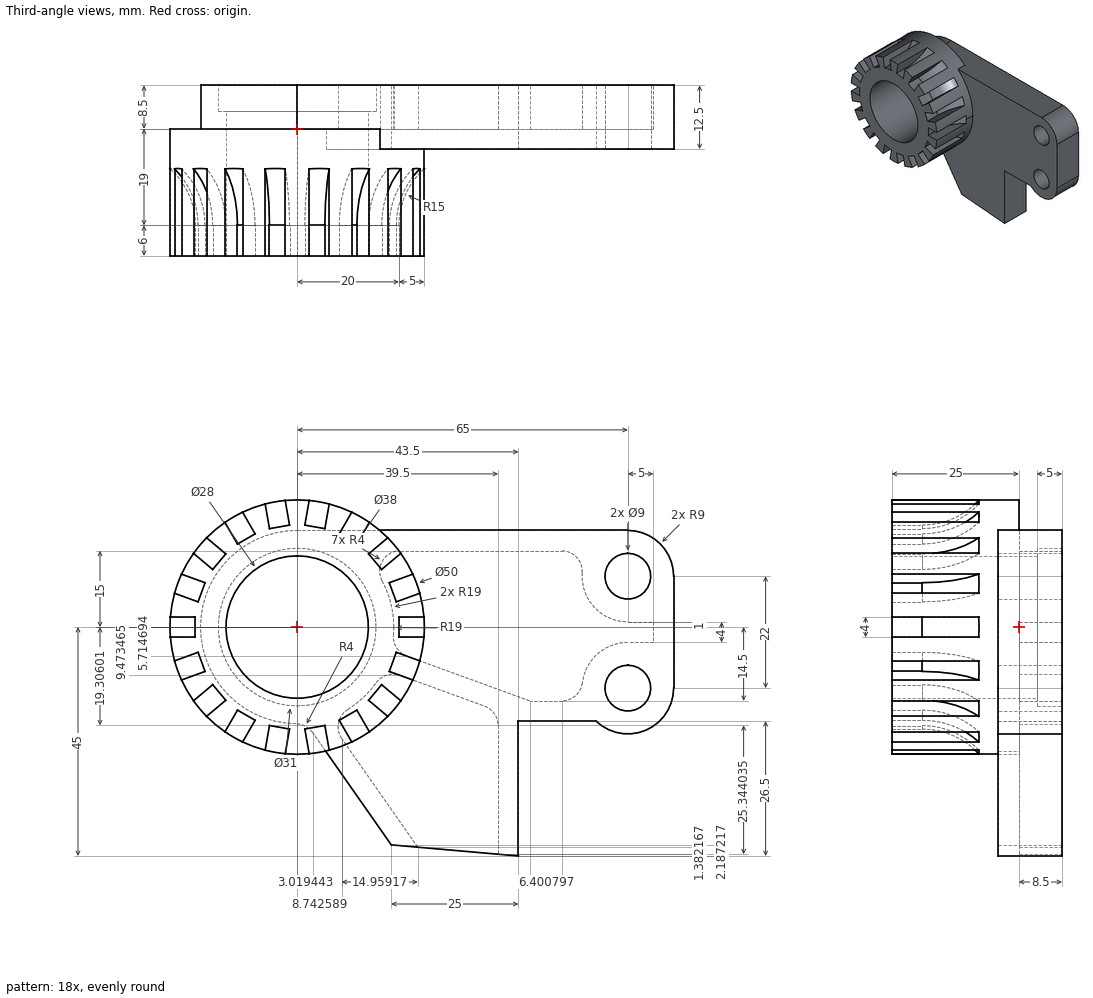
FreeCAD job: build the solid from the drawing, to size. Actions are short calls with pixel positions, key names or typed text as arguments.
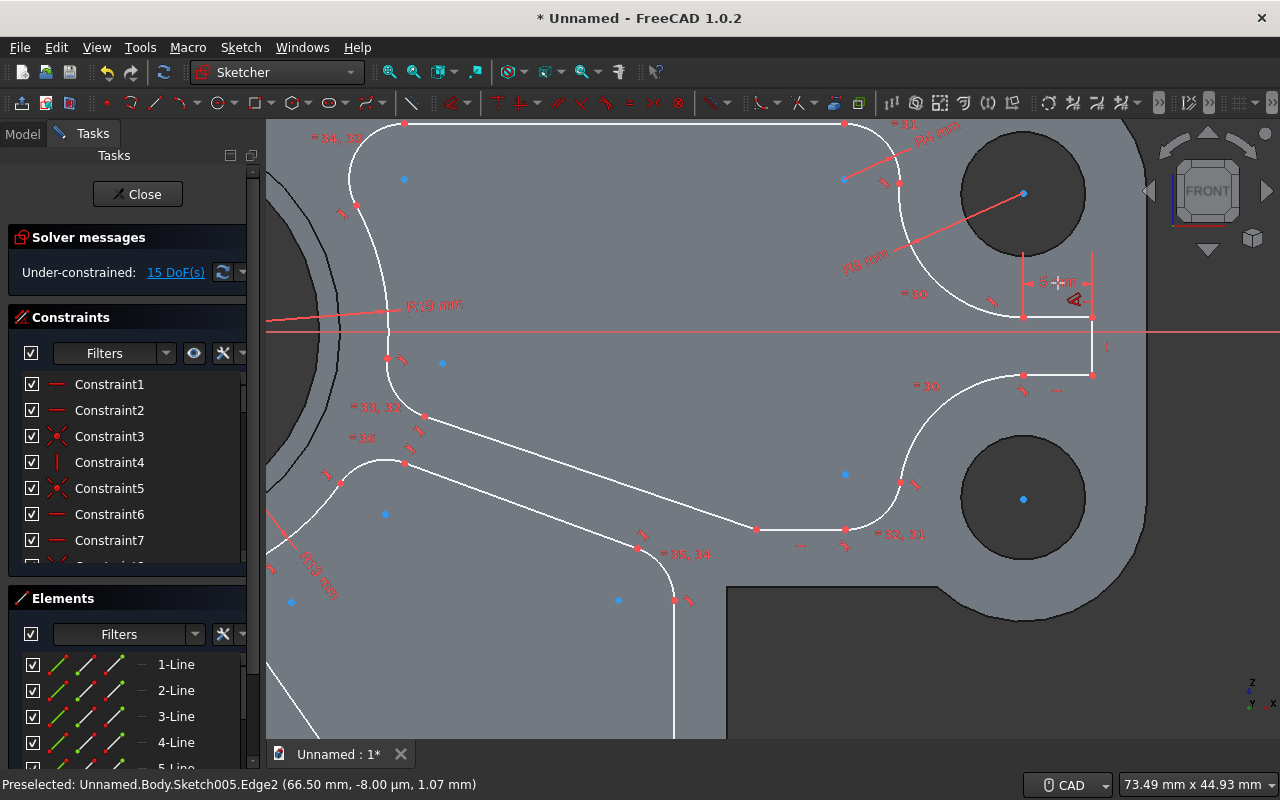
click(1092, 335)
click(1058, 346)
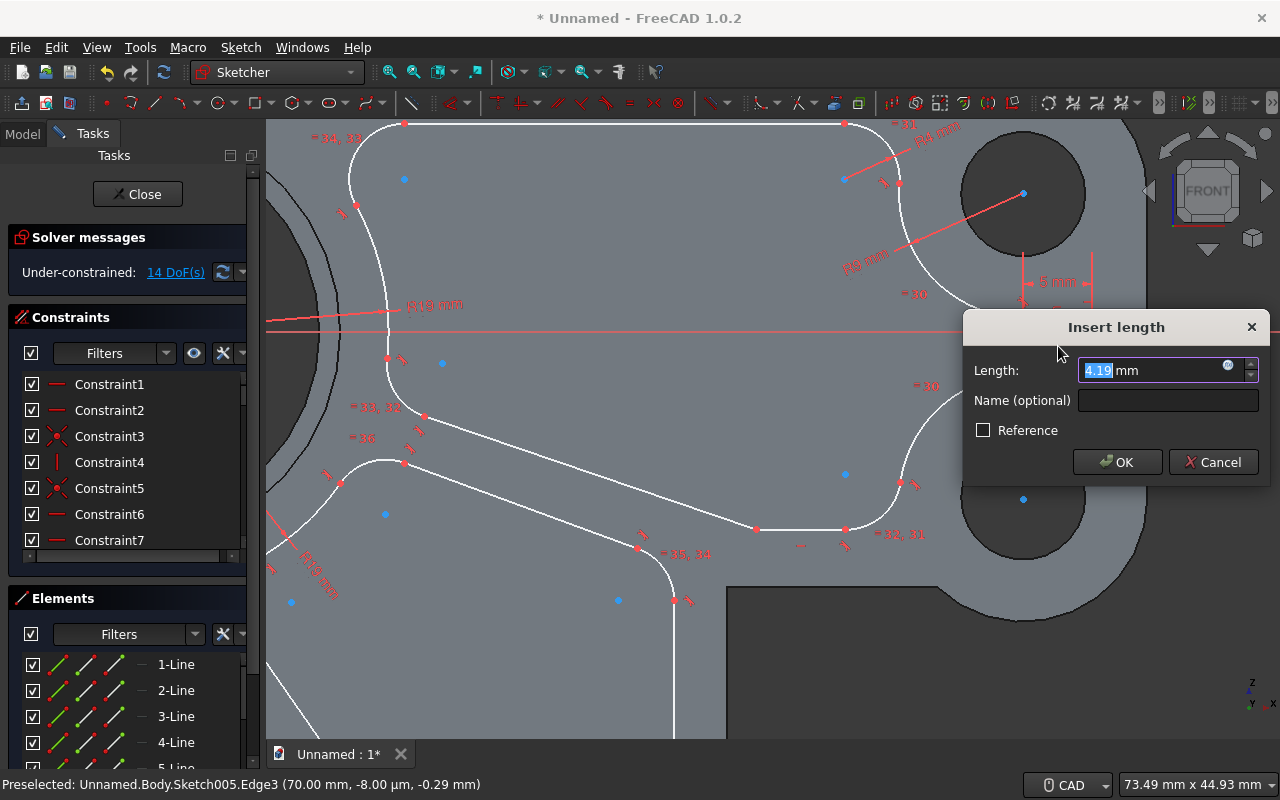
text(4)
key(Return)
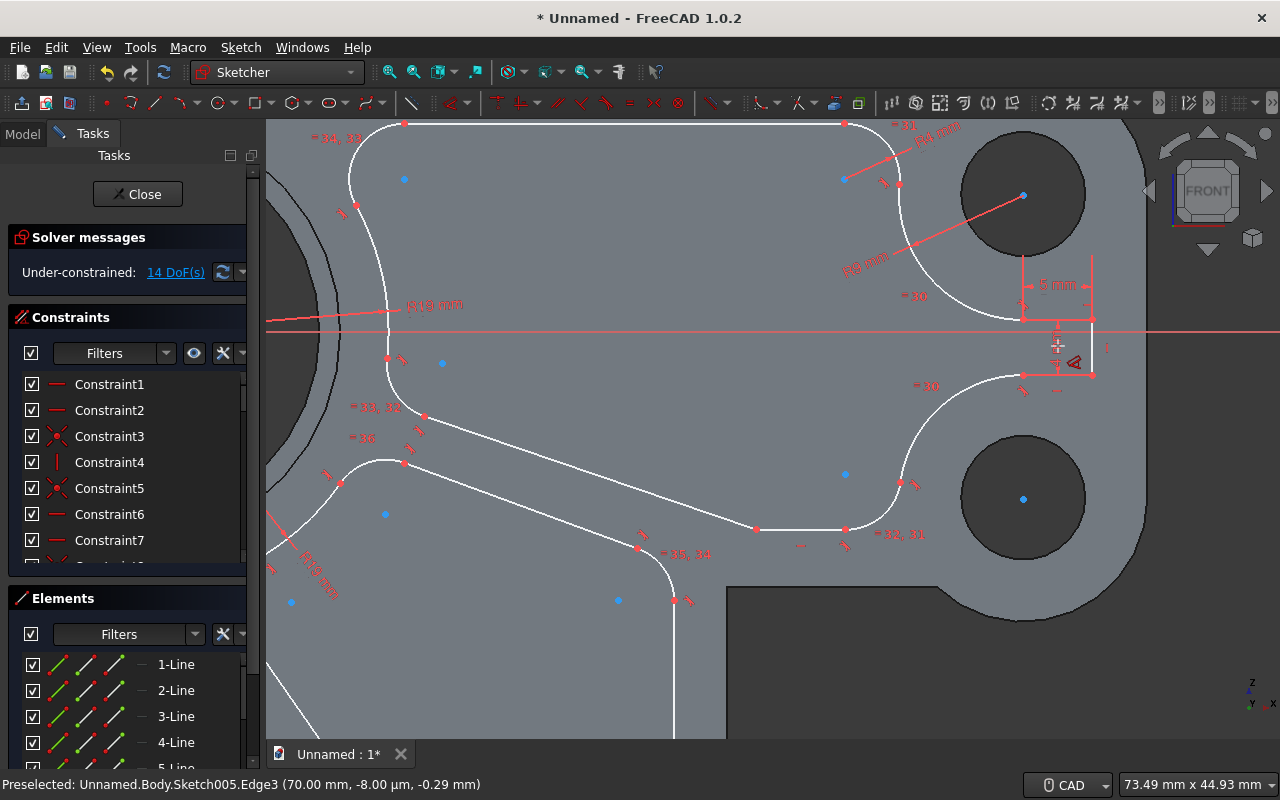
click(1072, 375)
click(1058, 409)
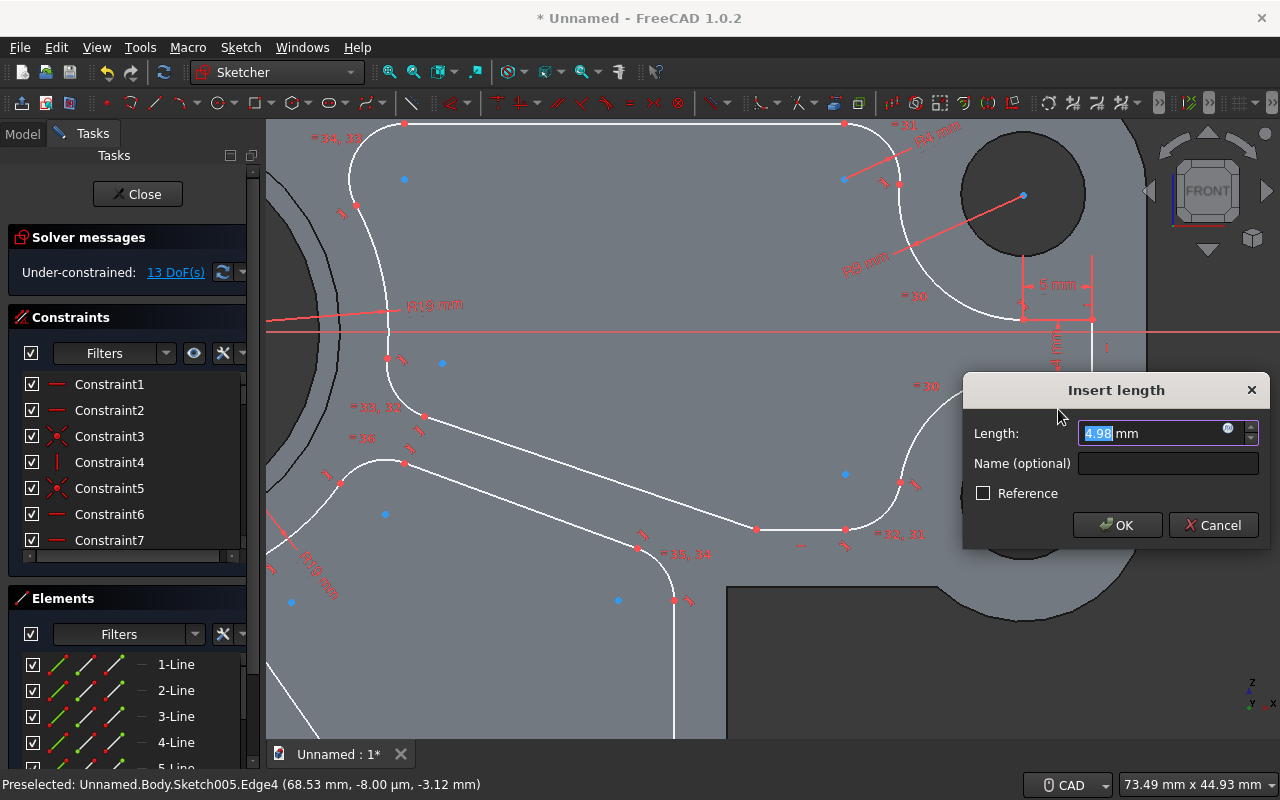
text(5)
key(Return)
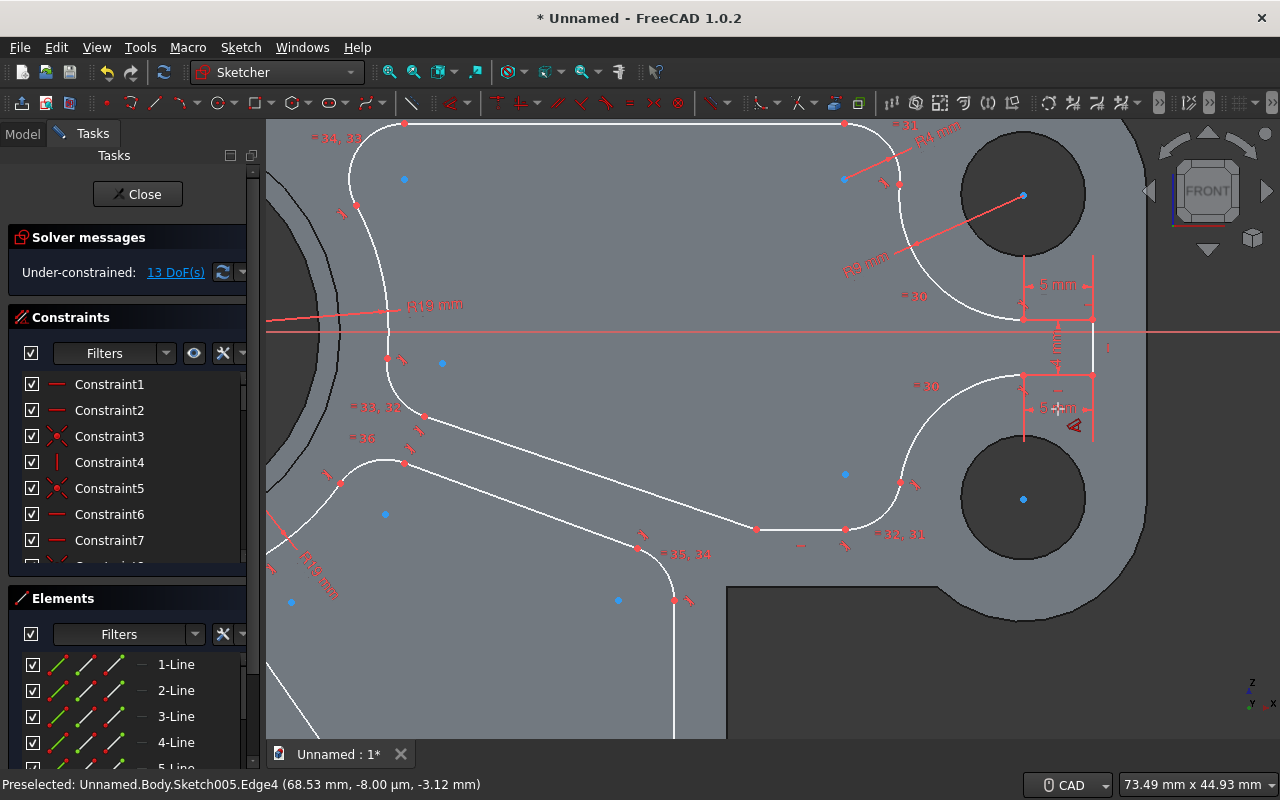
scroll(1024, 320, up, 6)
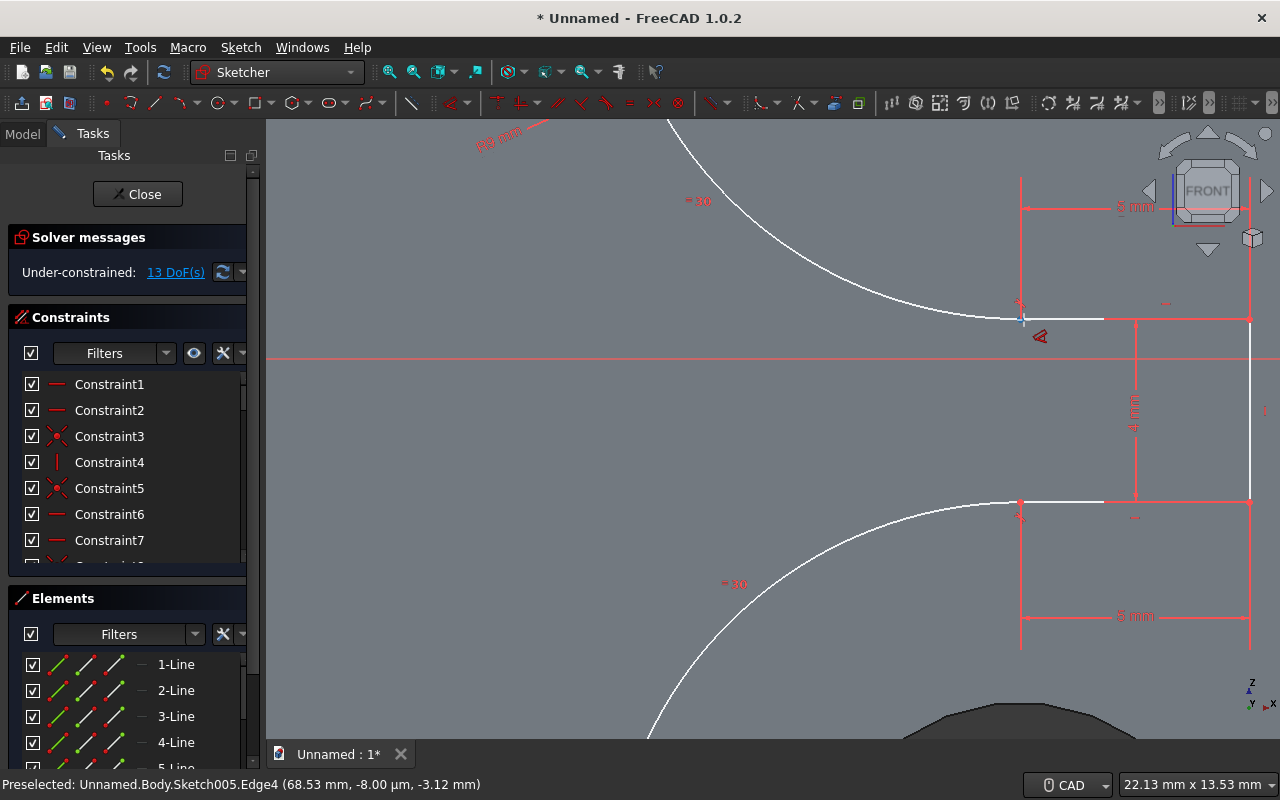
click(1021, 319)
click(1055, 339)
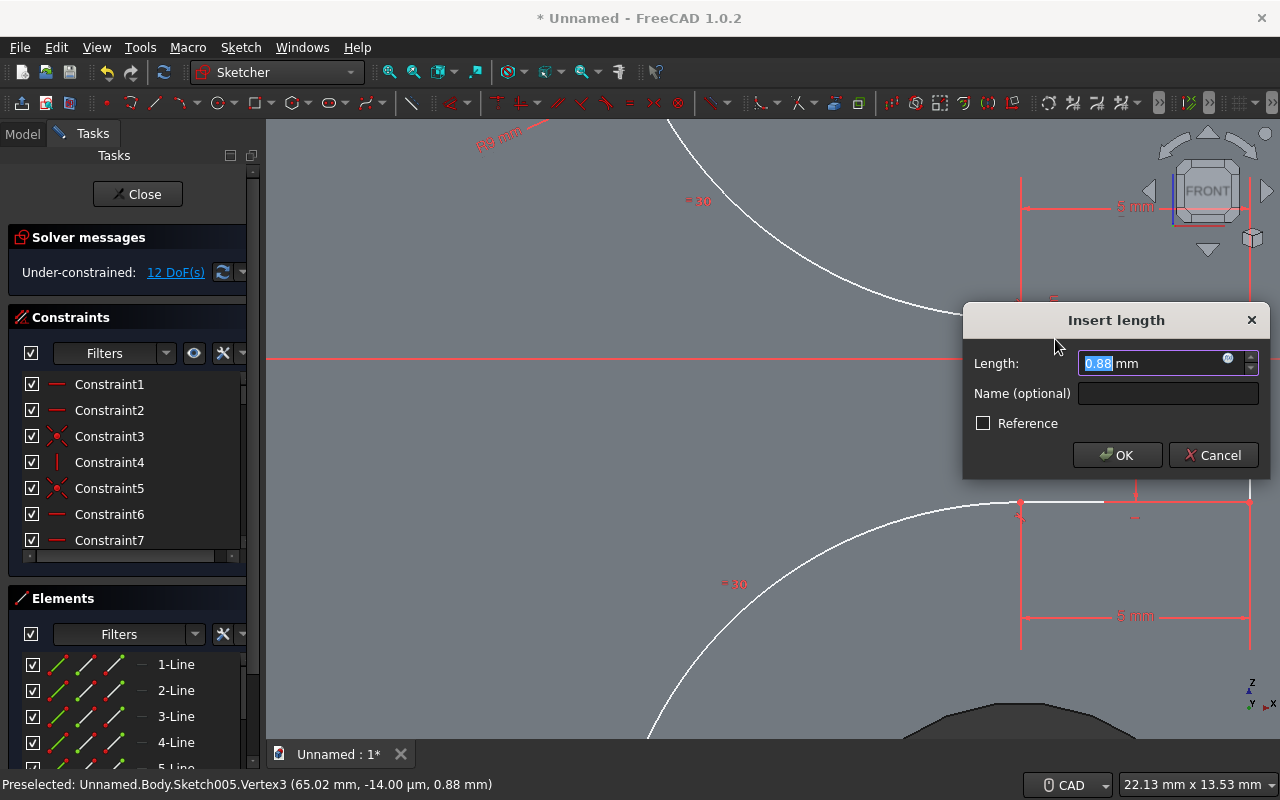
text(1)
key(Return)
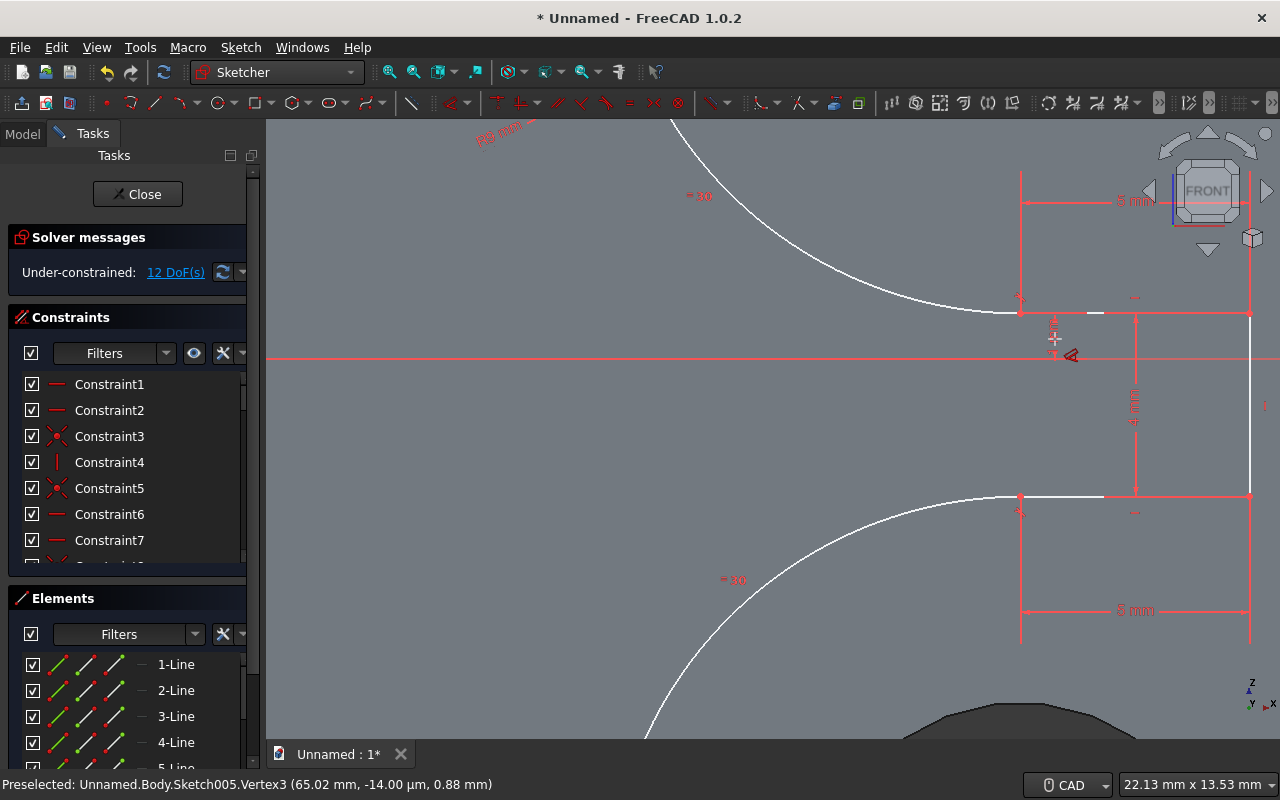
scroll(870, 334, down, 10)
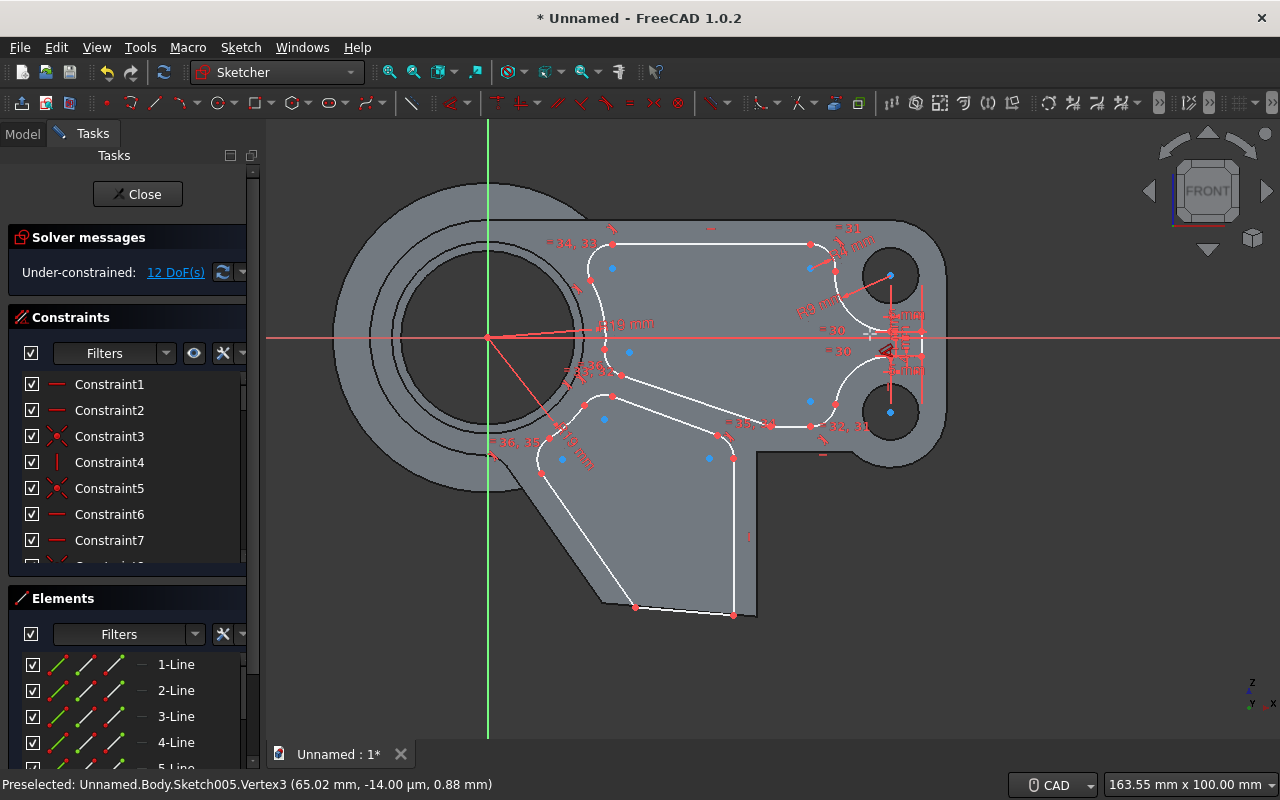
click(613, 244)
click(454, 291)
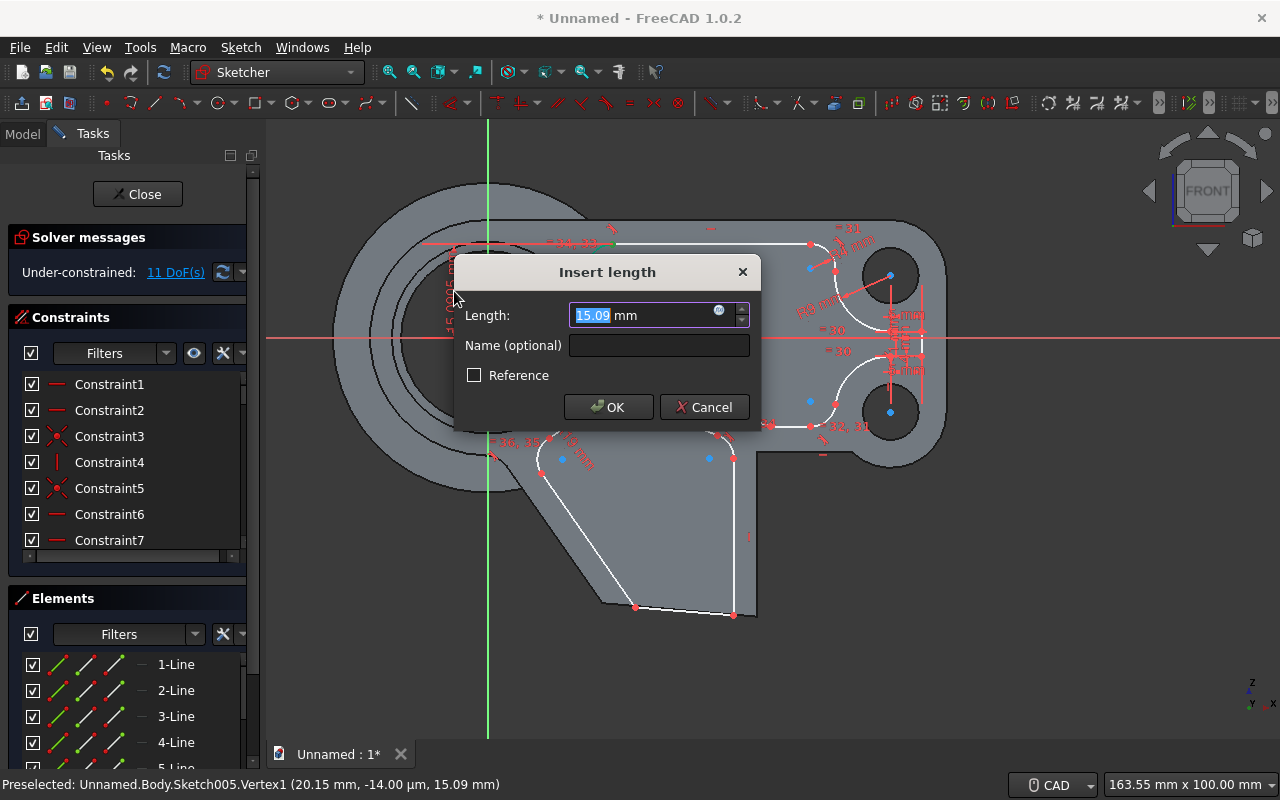
text(15)
key(Return)